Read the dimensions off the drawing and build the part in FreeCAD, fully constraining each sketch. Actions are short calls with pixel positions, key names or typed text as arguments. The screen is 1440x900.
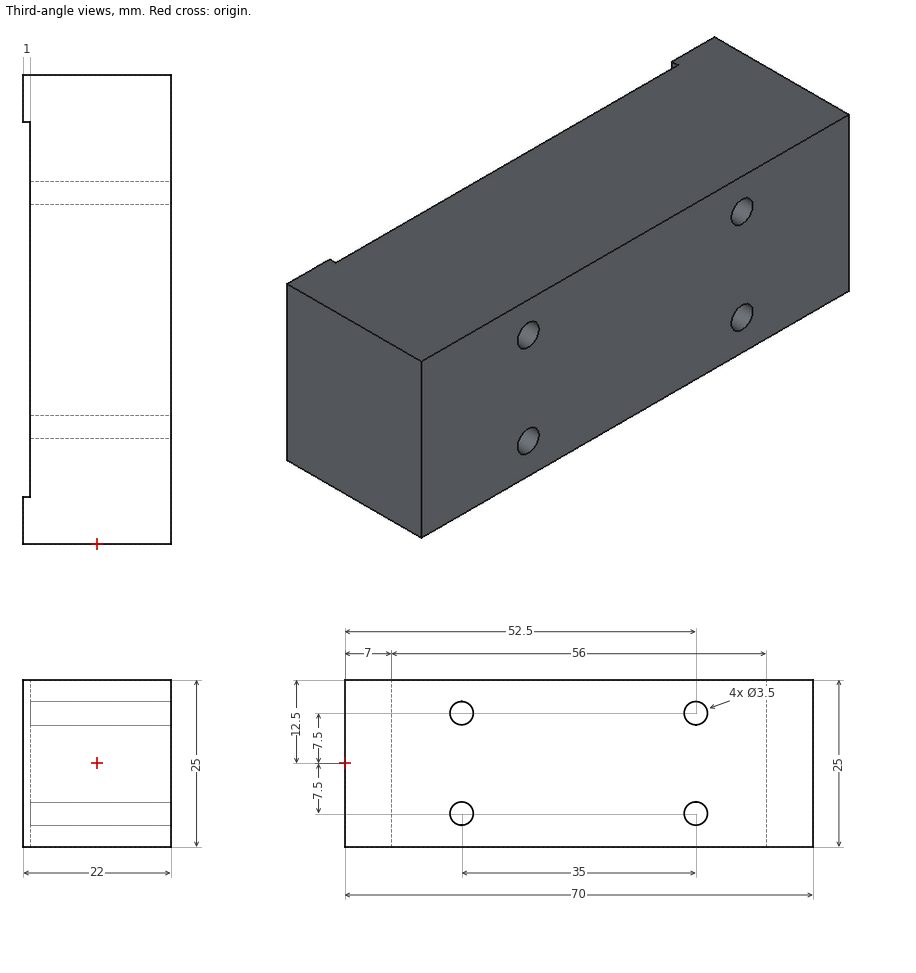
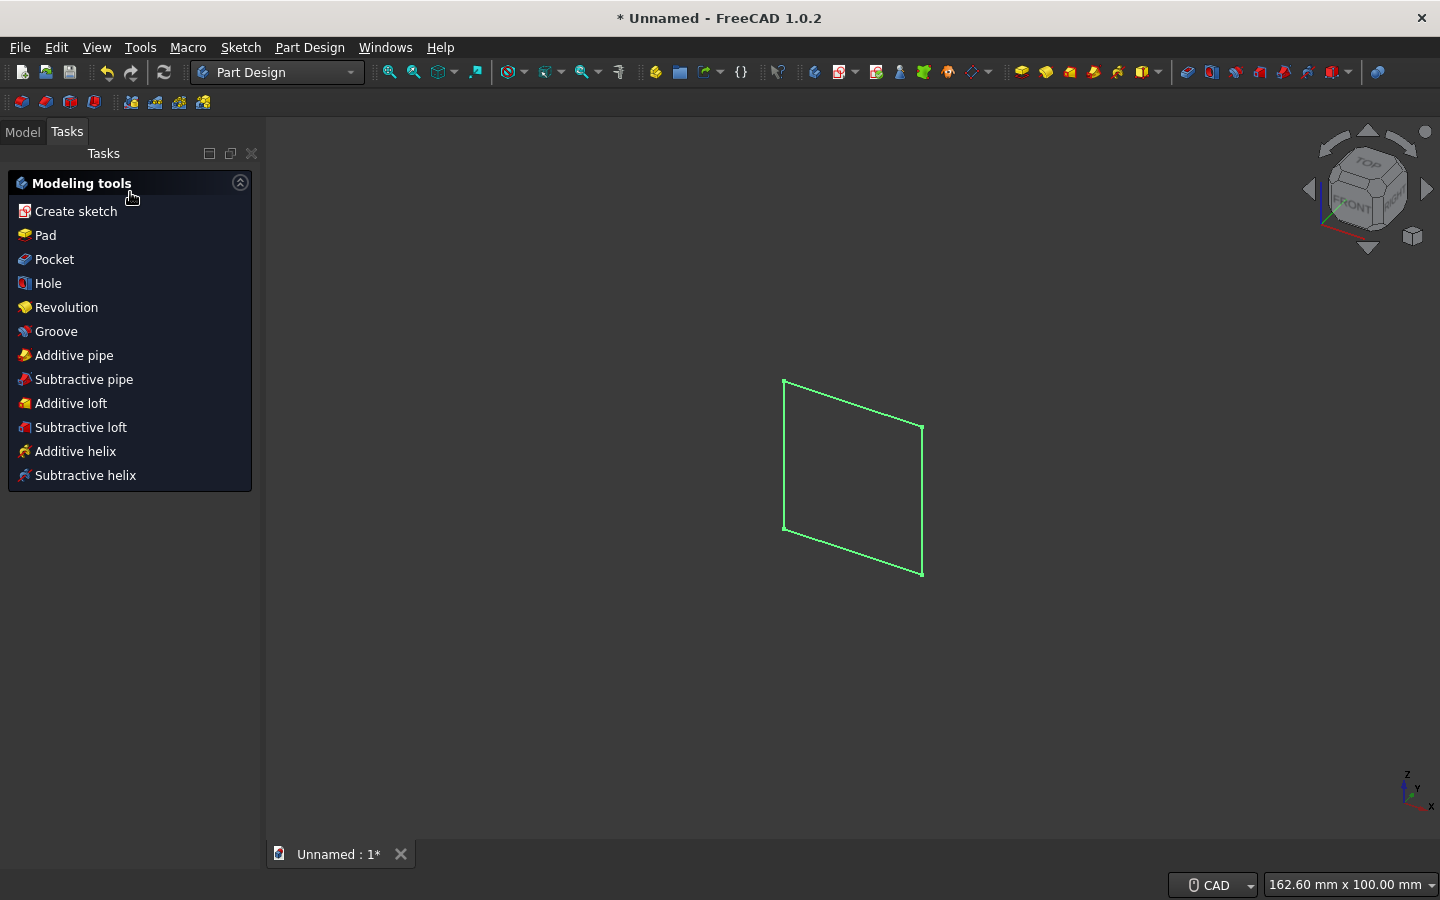
click(1022, 72)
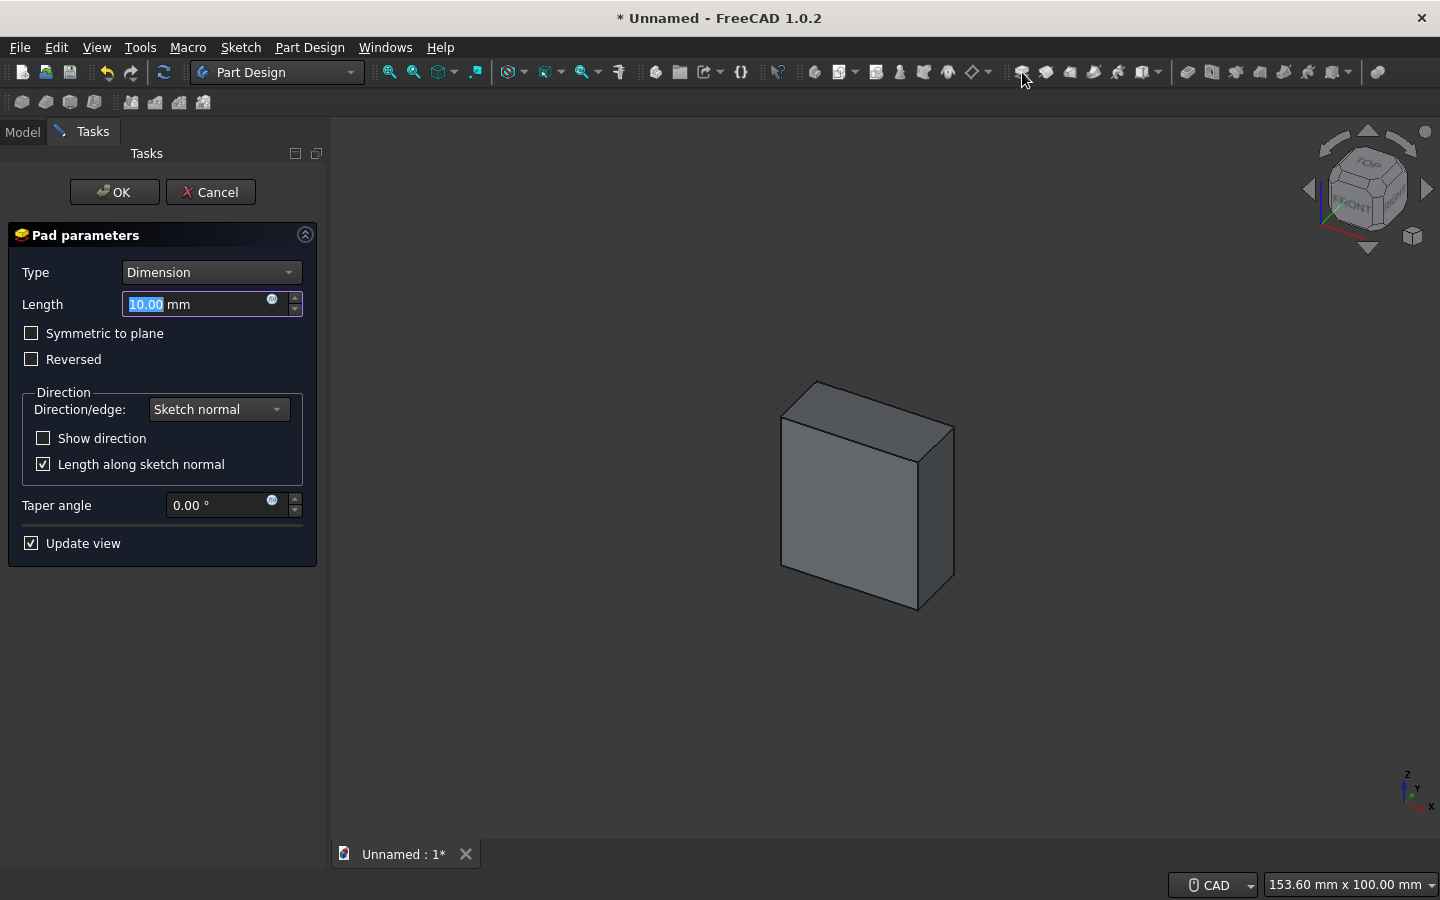
text(70)
key(Tab)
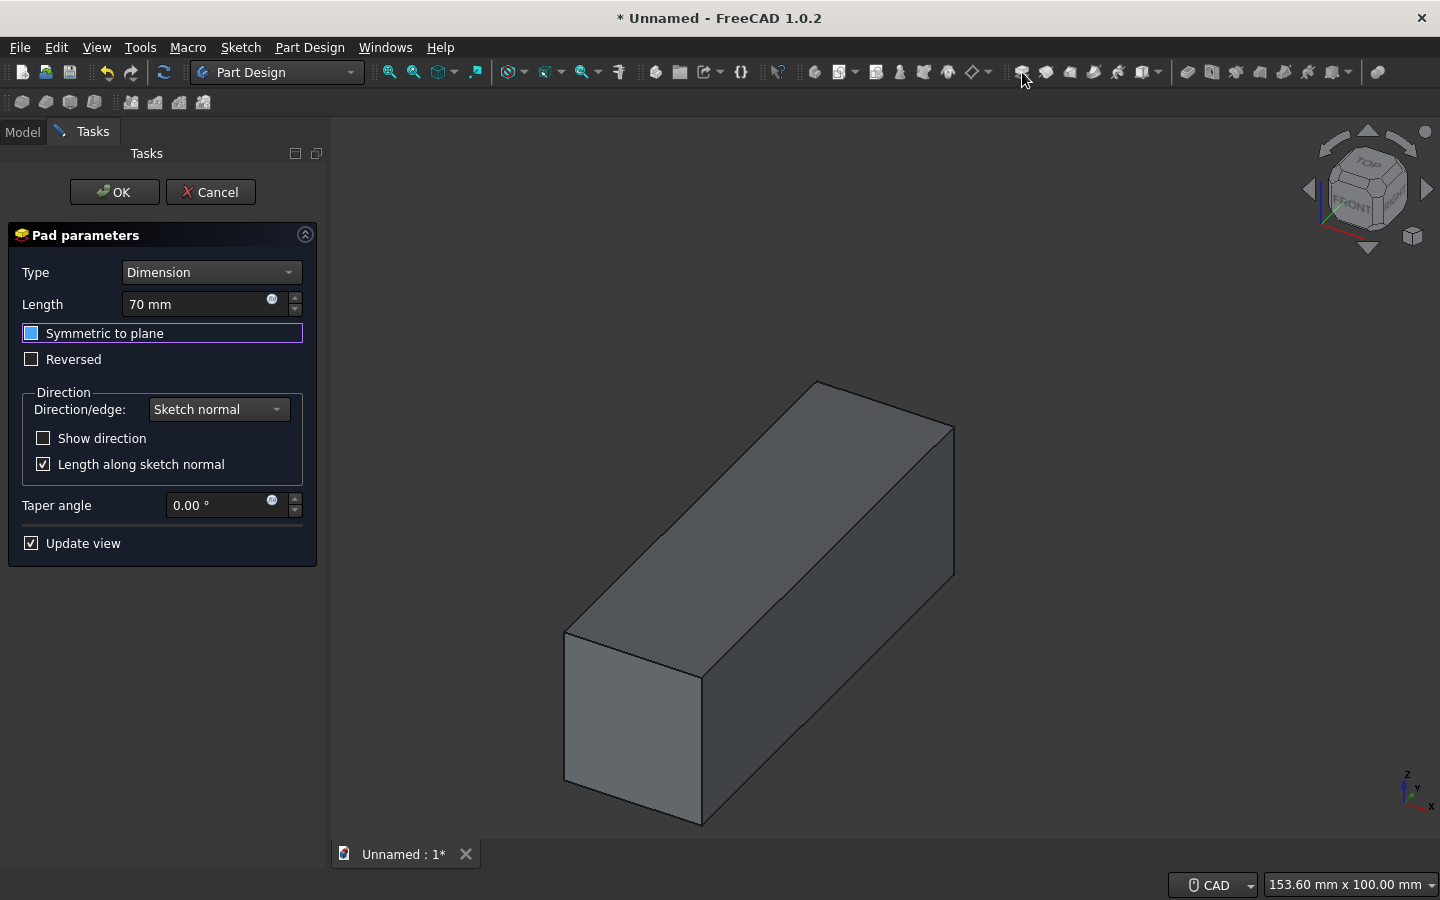
click(30, 359)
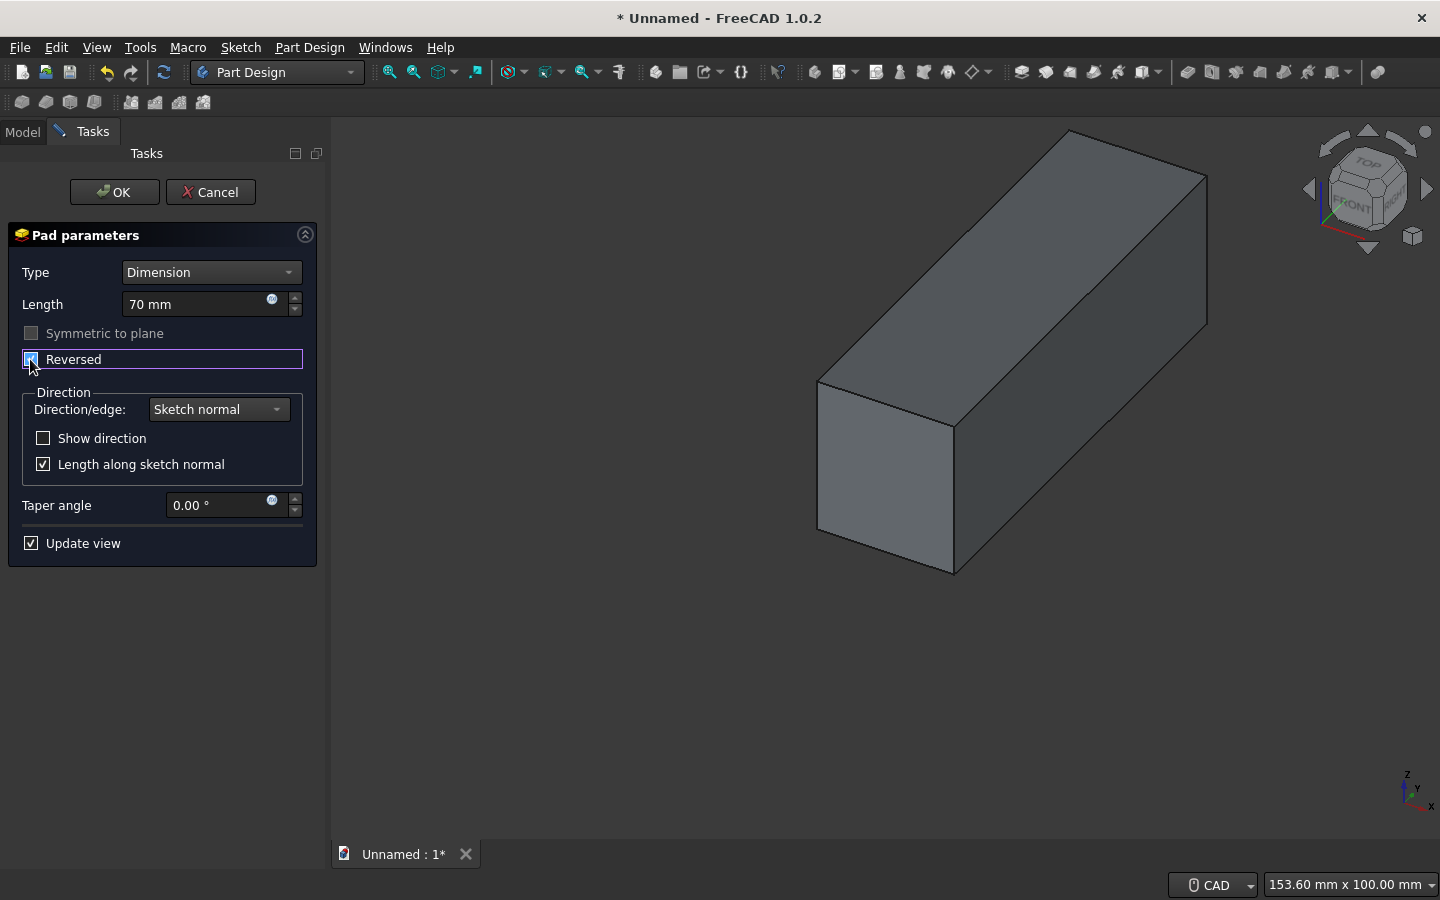
click(115, 192)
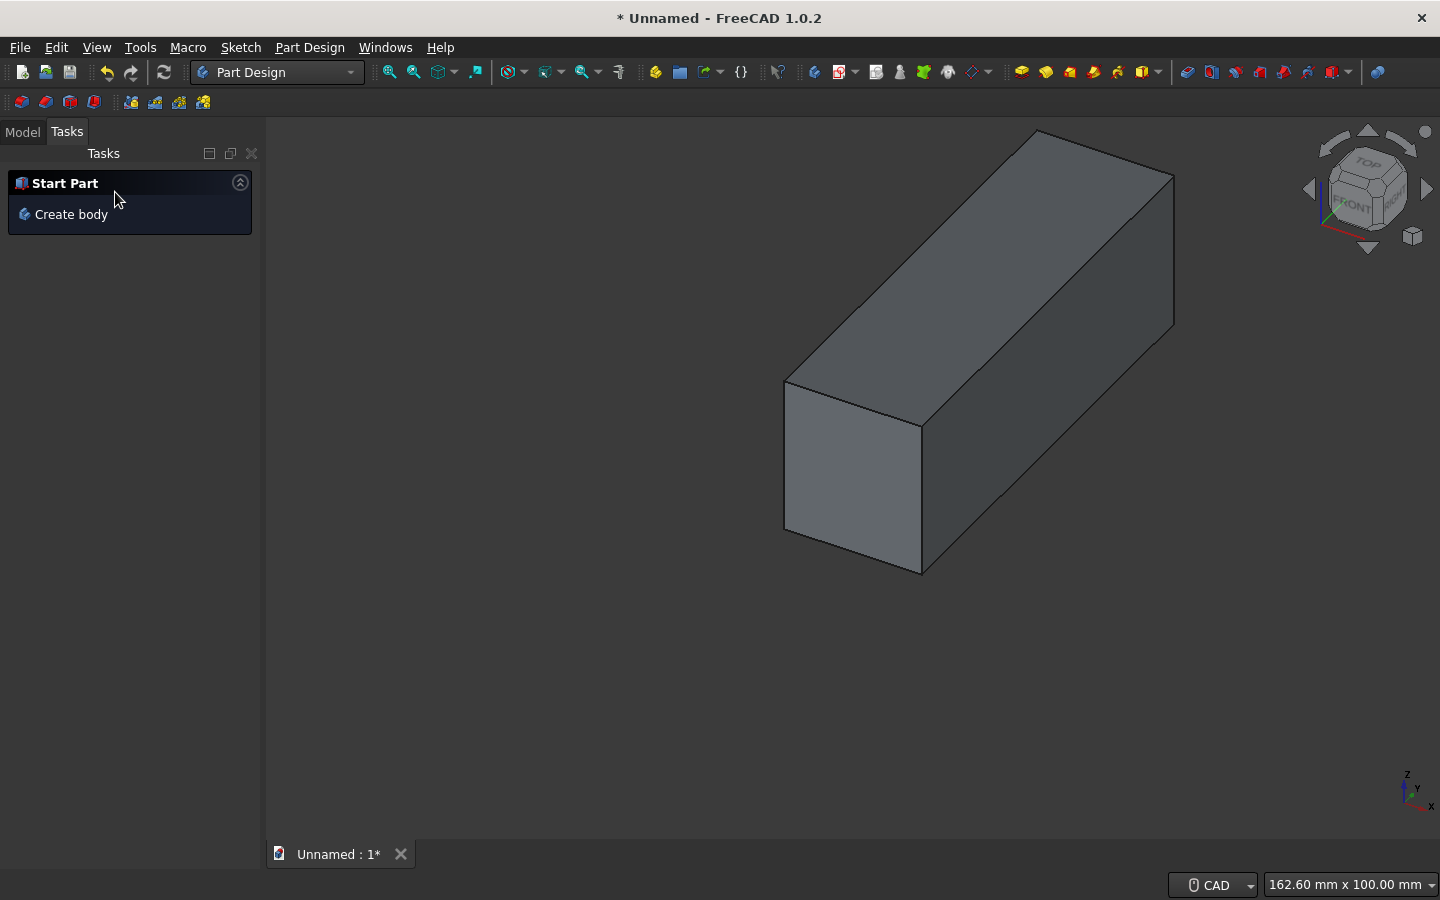
click(1120, 303)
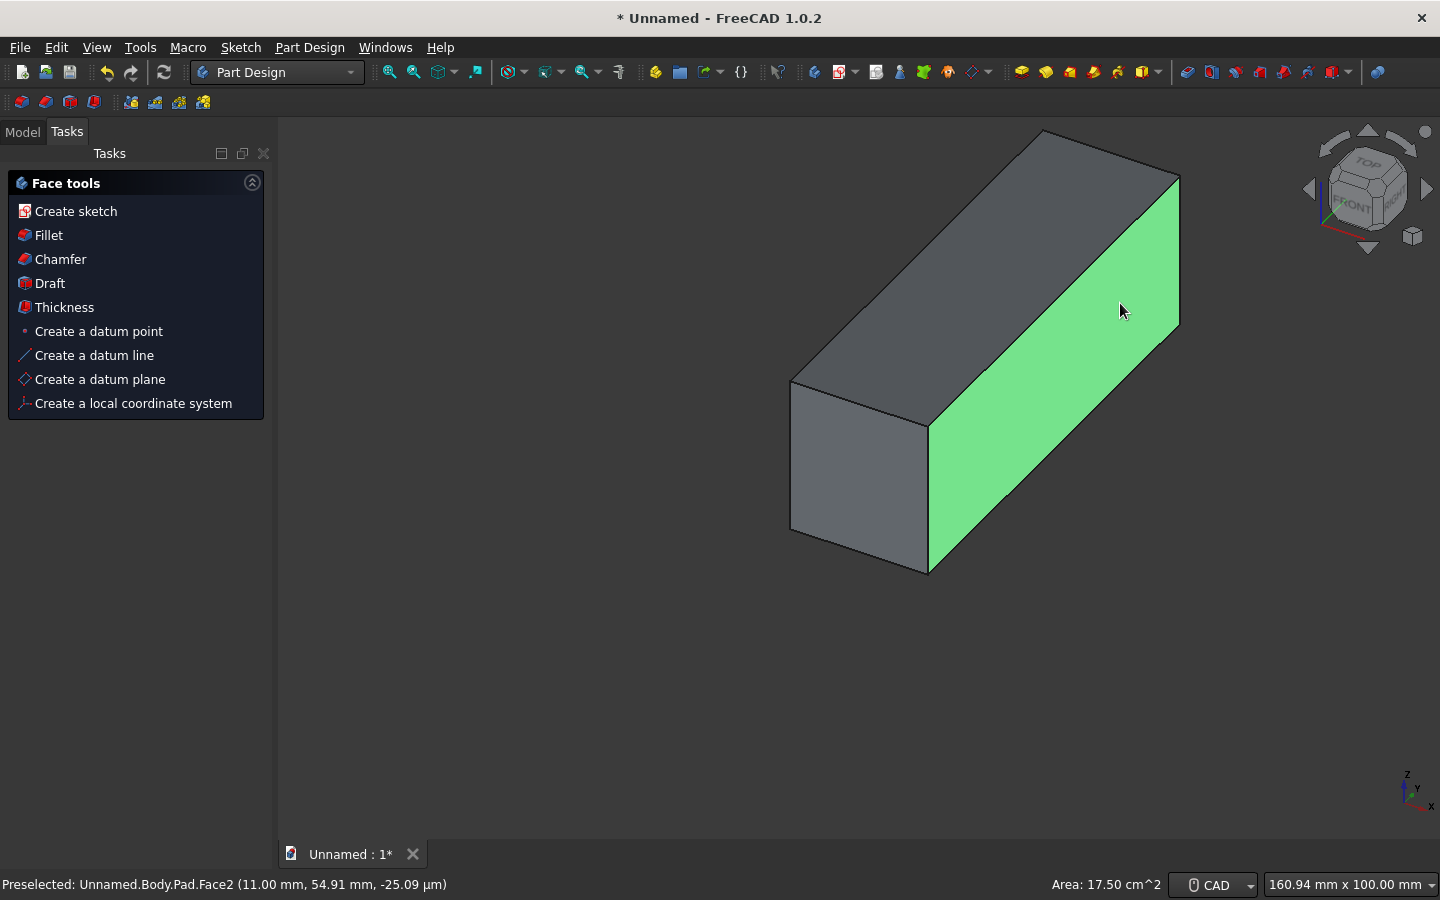
click(840, 72)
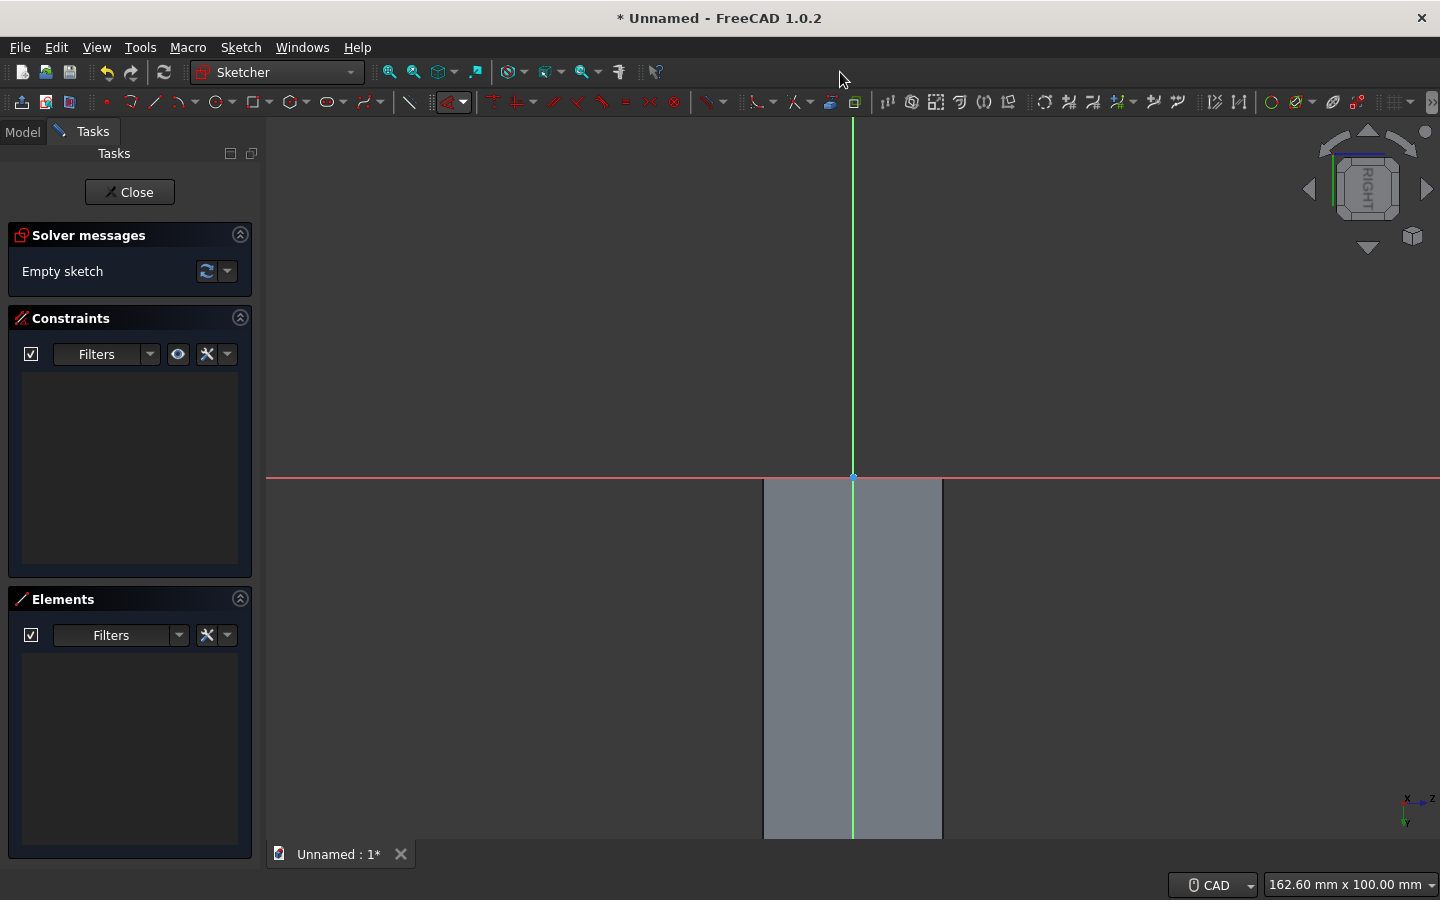
scroll(475, 145, down, 1)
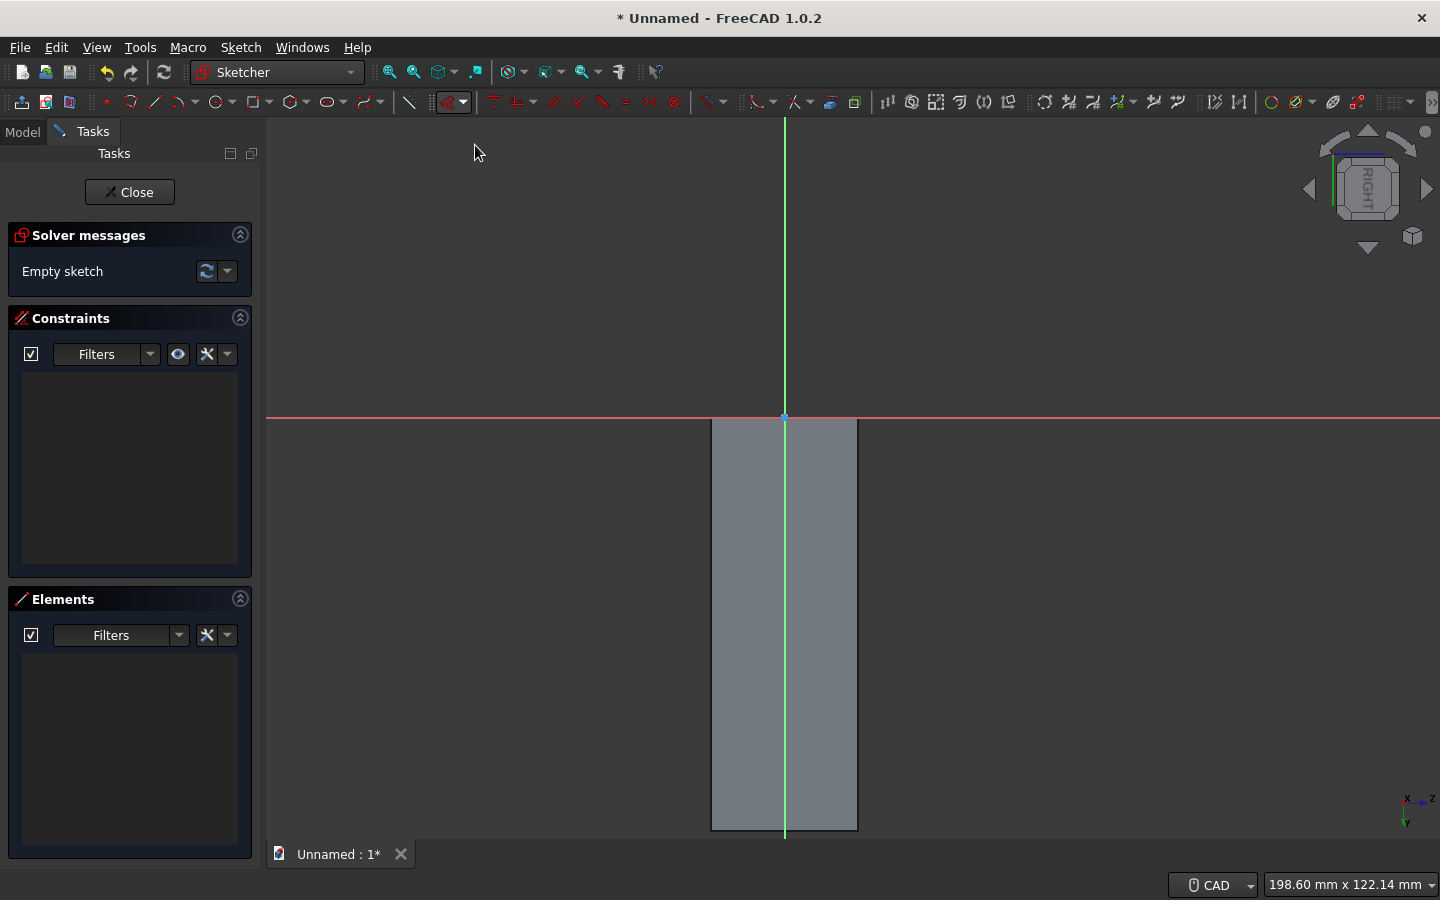
scroll(785, 781, up, 2)